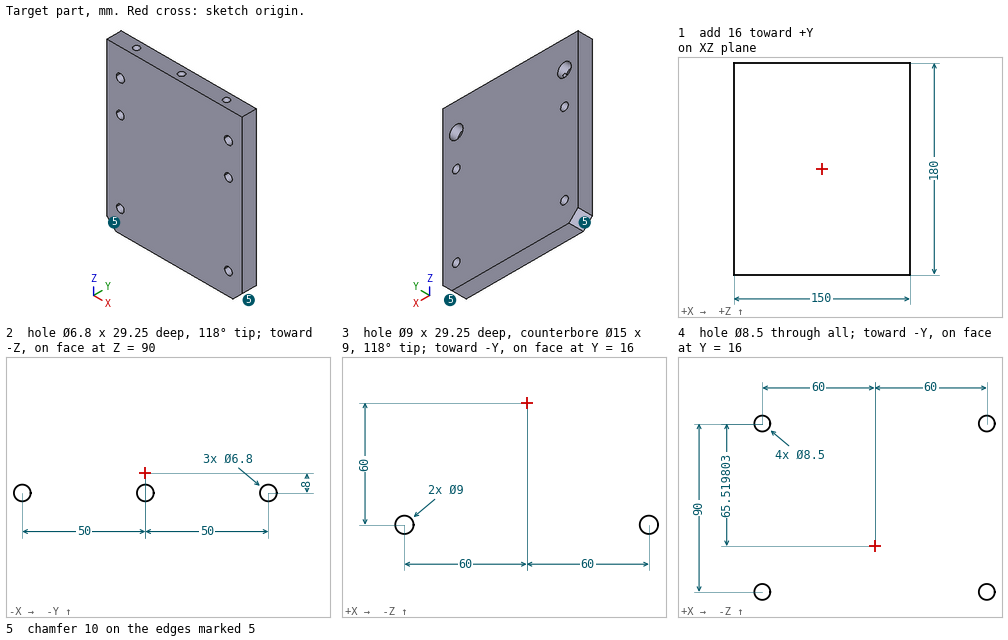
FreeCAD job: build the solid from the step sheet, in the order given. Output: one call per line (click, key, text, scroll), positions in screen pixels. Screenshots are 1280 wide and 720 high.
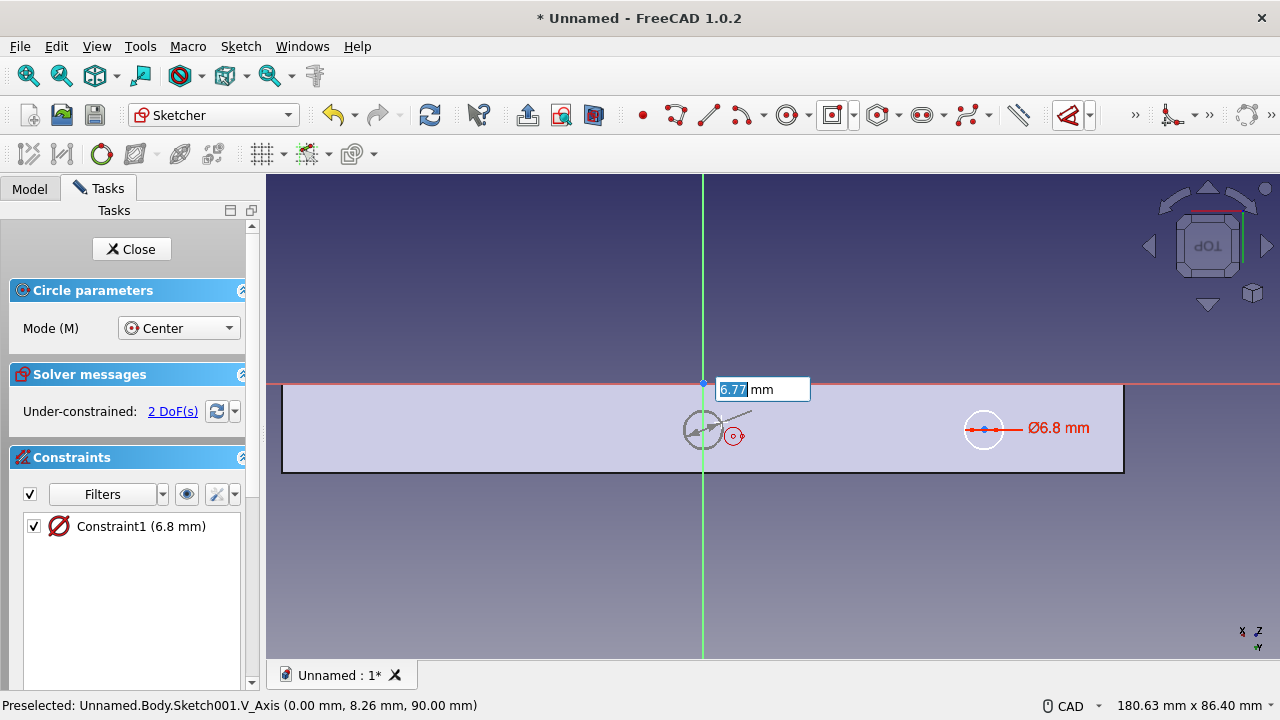
text(6.8)
key(Return)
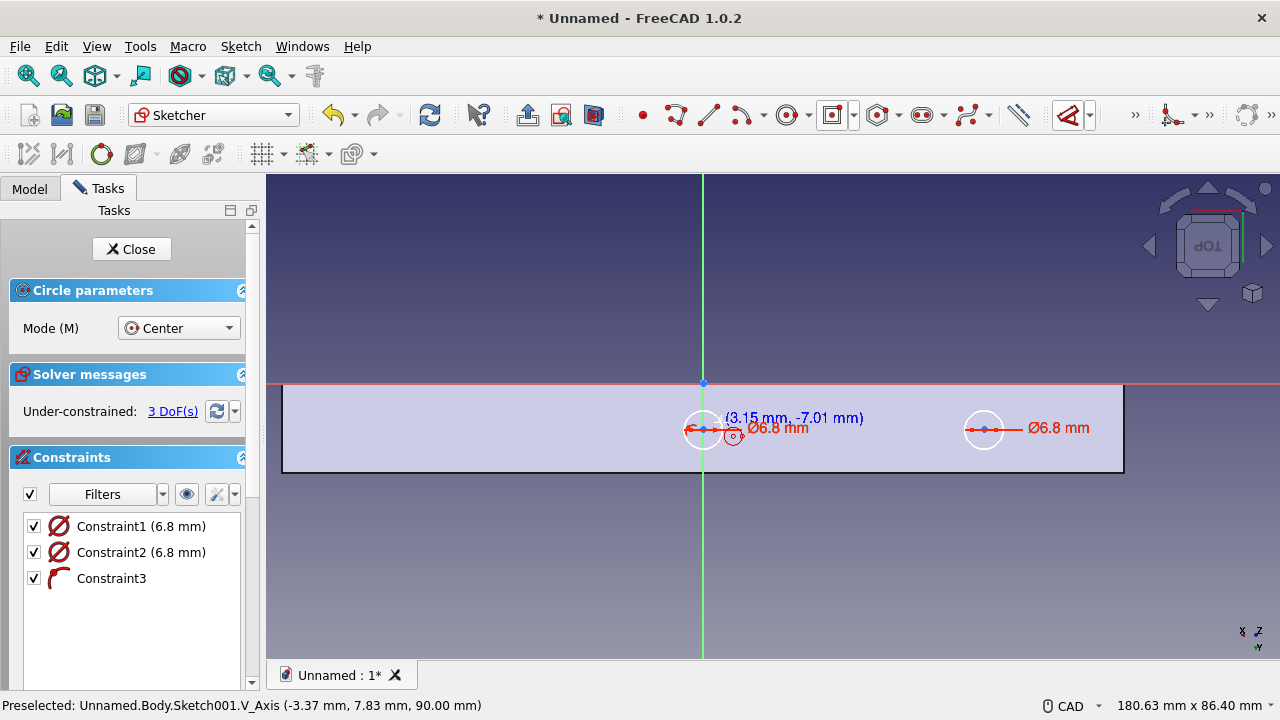
click(423, 429)
move(436, 415)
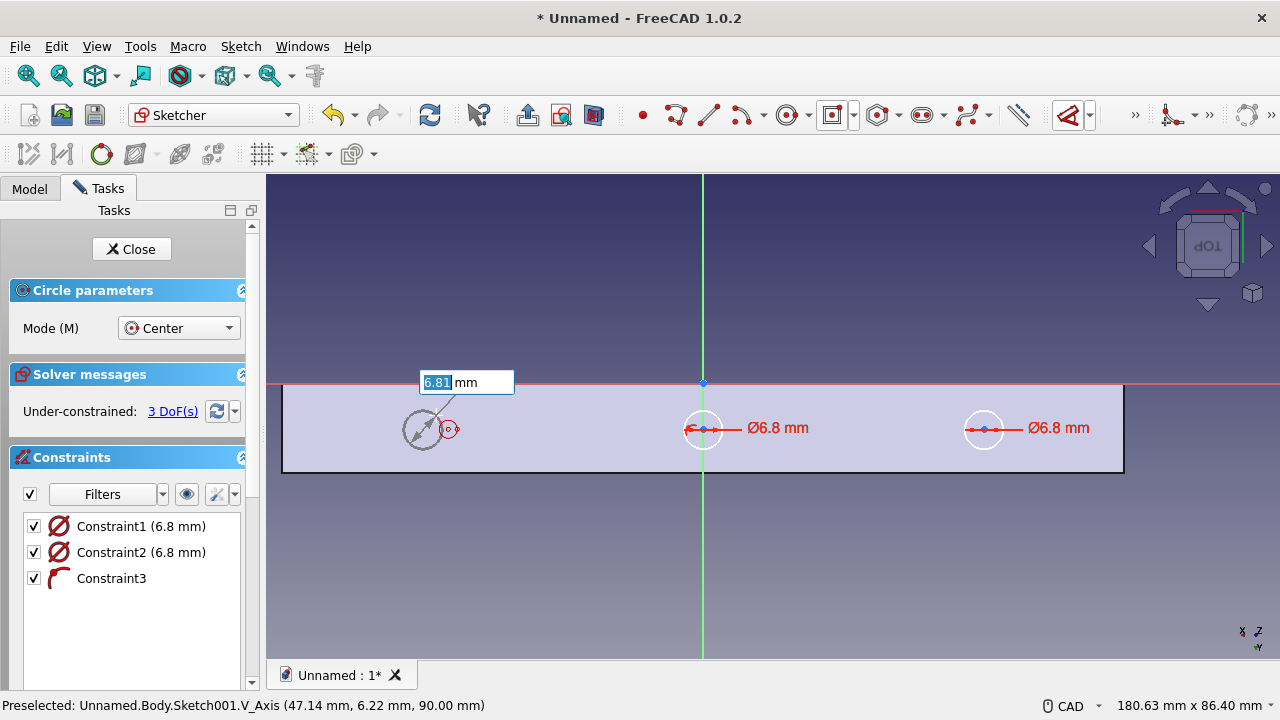
text(6.8)
key(Return)
key(Escape)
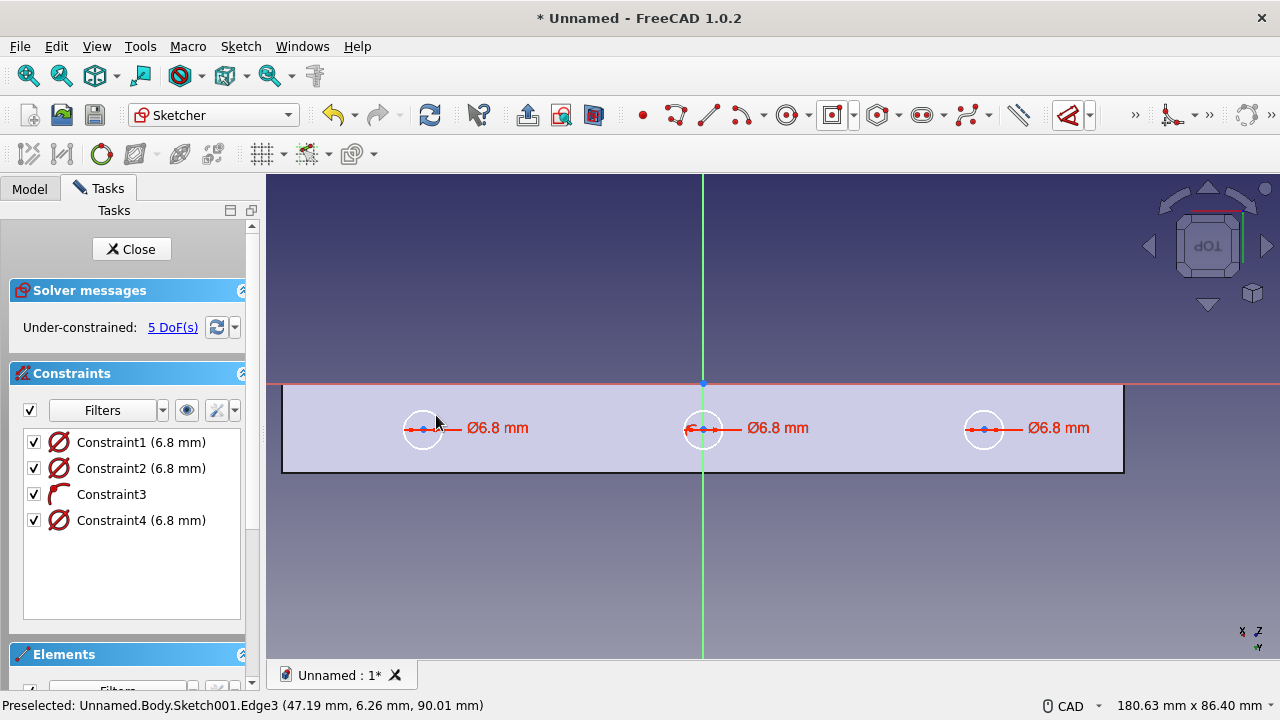
click(984, 430)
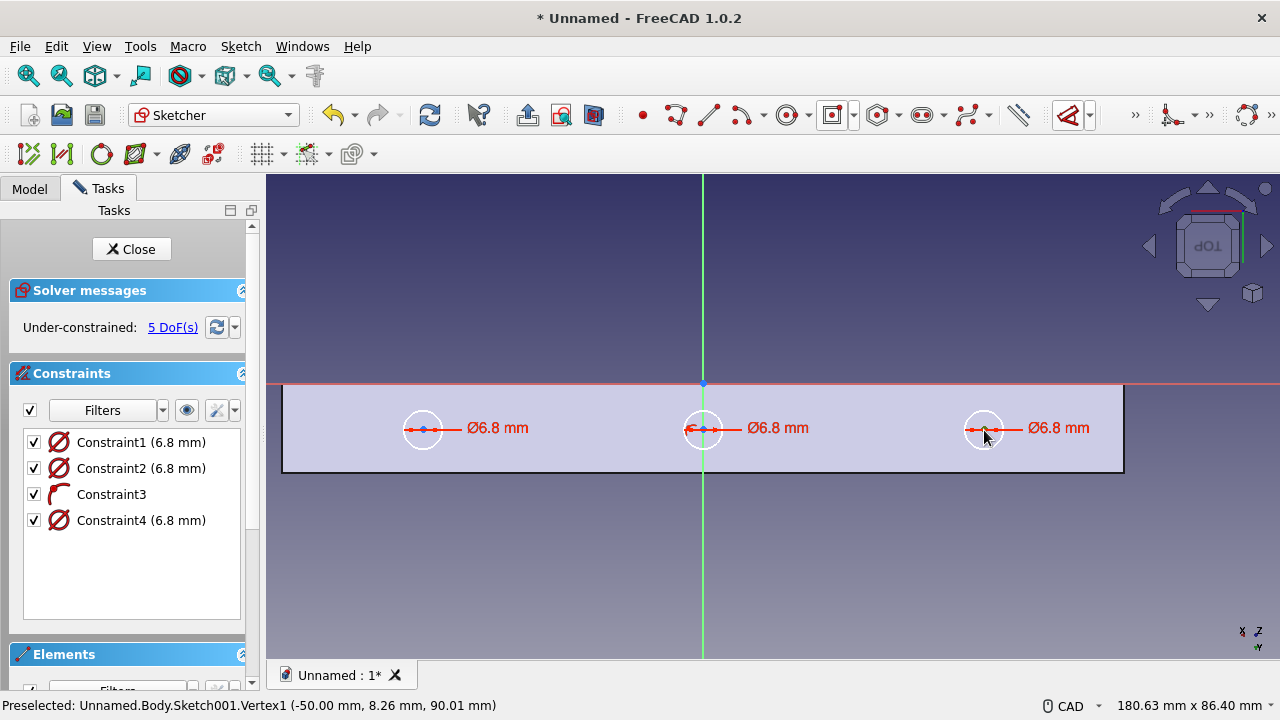
click(703, 430)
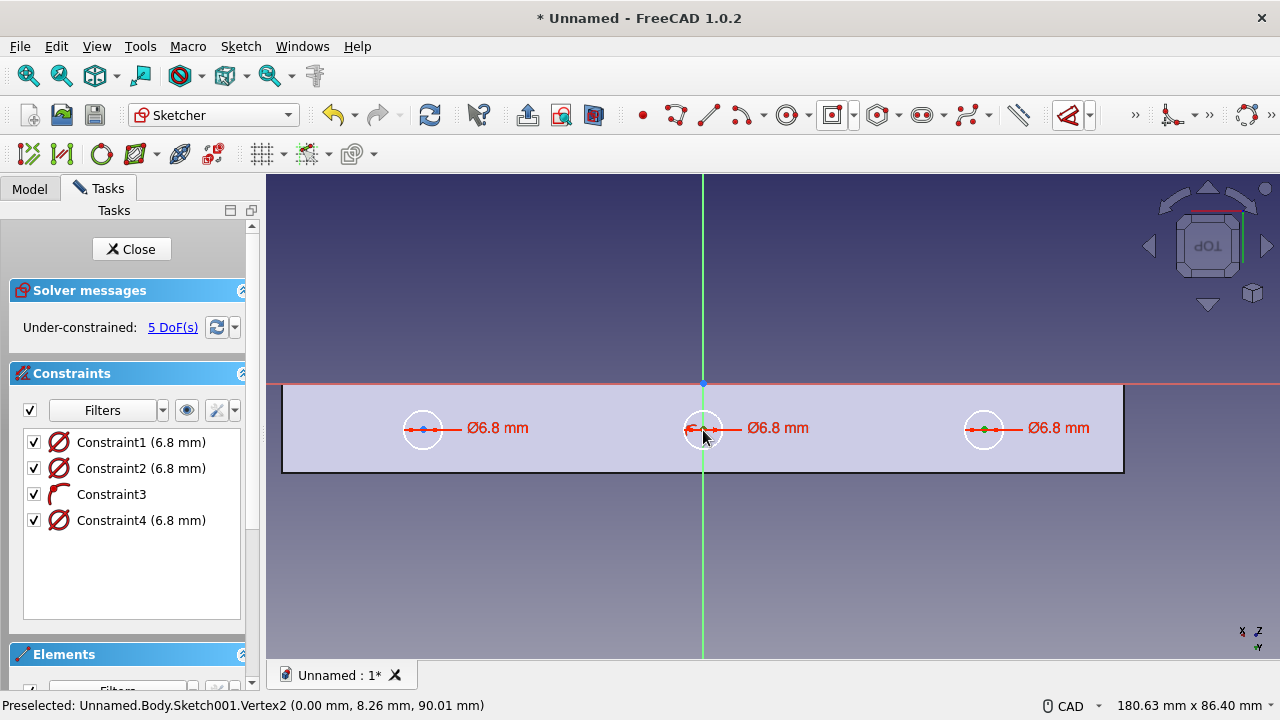
key(h)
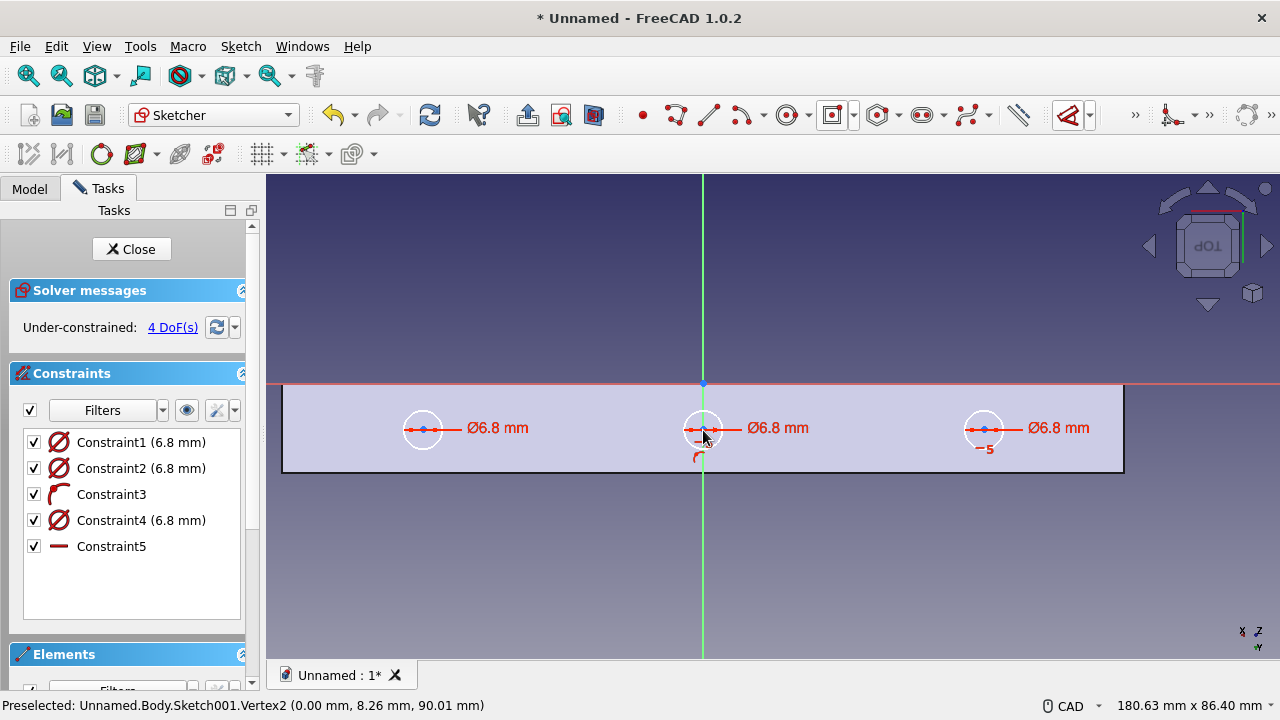
click(703, 430)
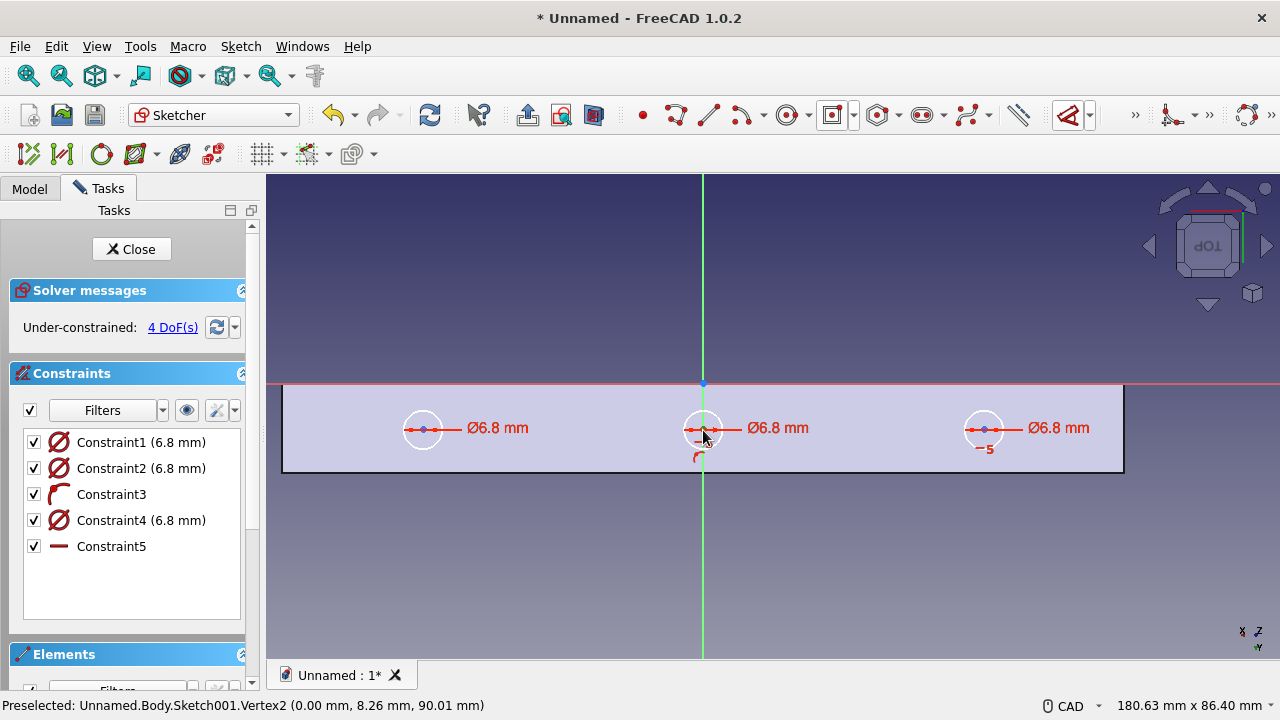
click(423, 430)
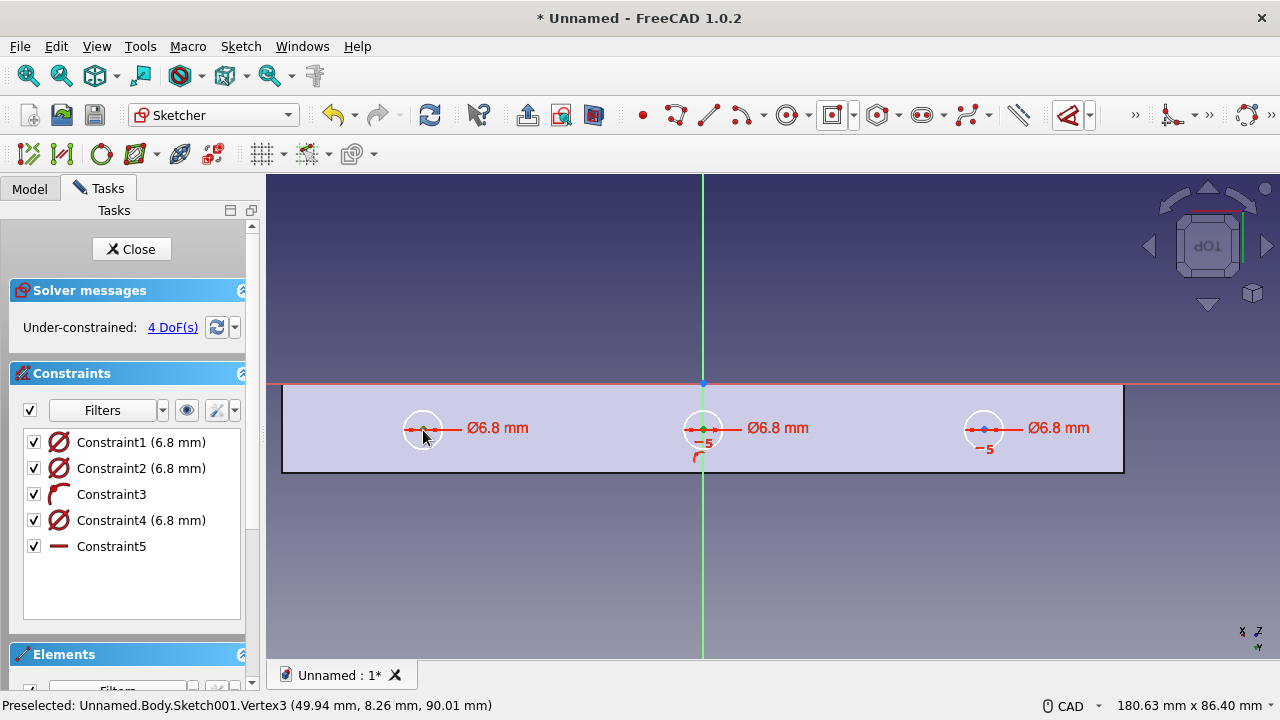
key(h)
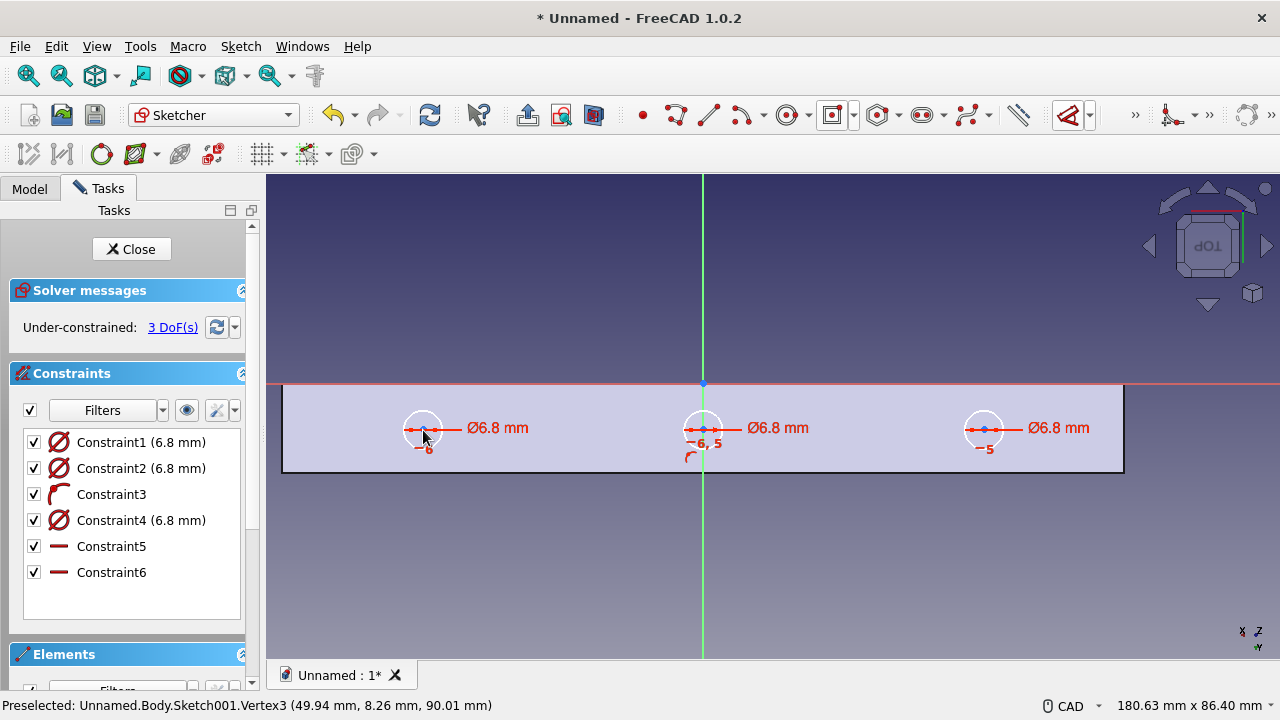
click(1068, 116)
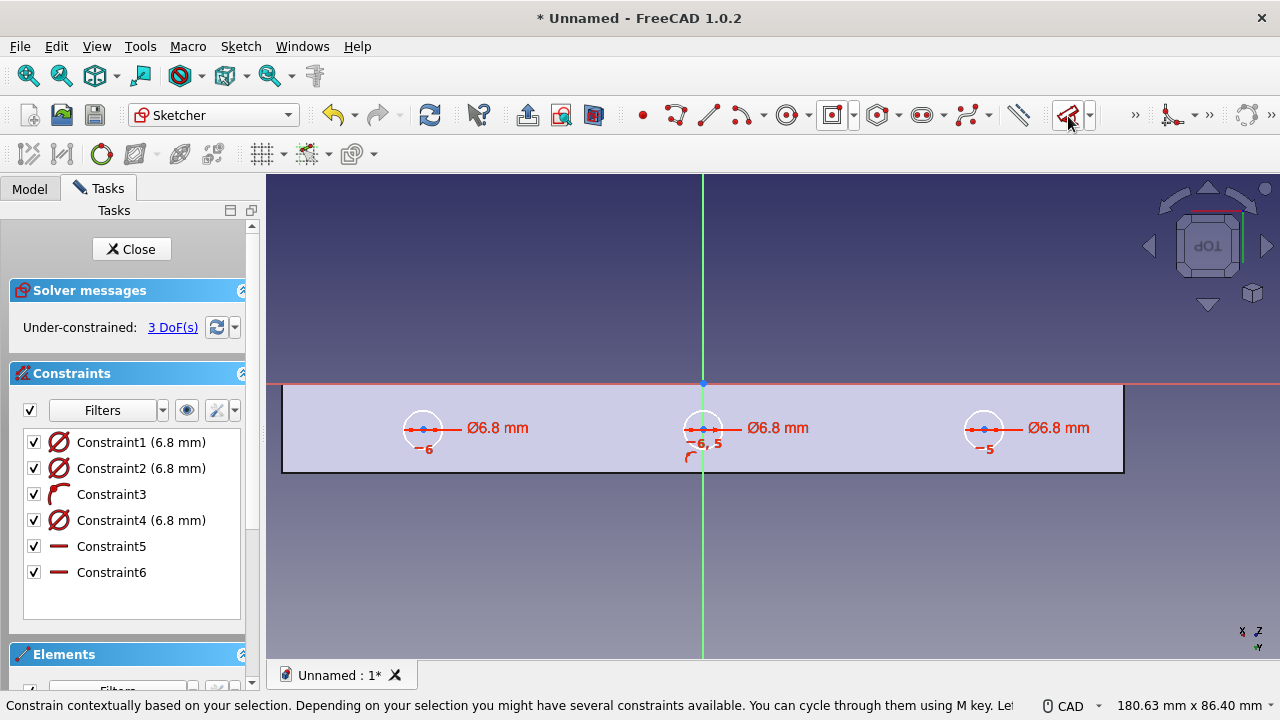
click(984, 430)
click(1018, 407)